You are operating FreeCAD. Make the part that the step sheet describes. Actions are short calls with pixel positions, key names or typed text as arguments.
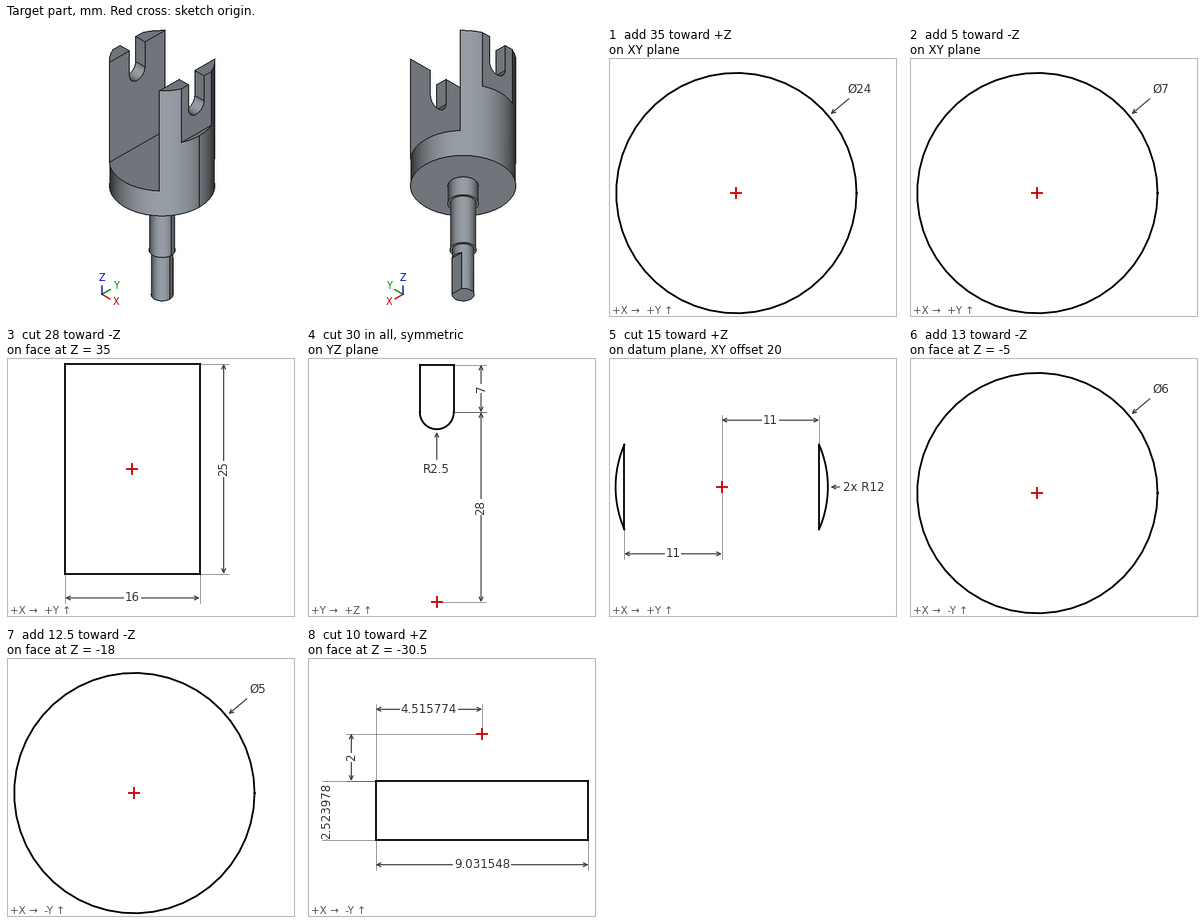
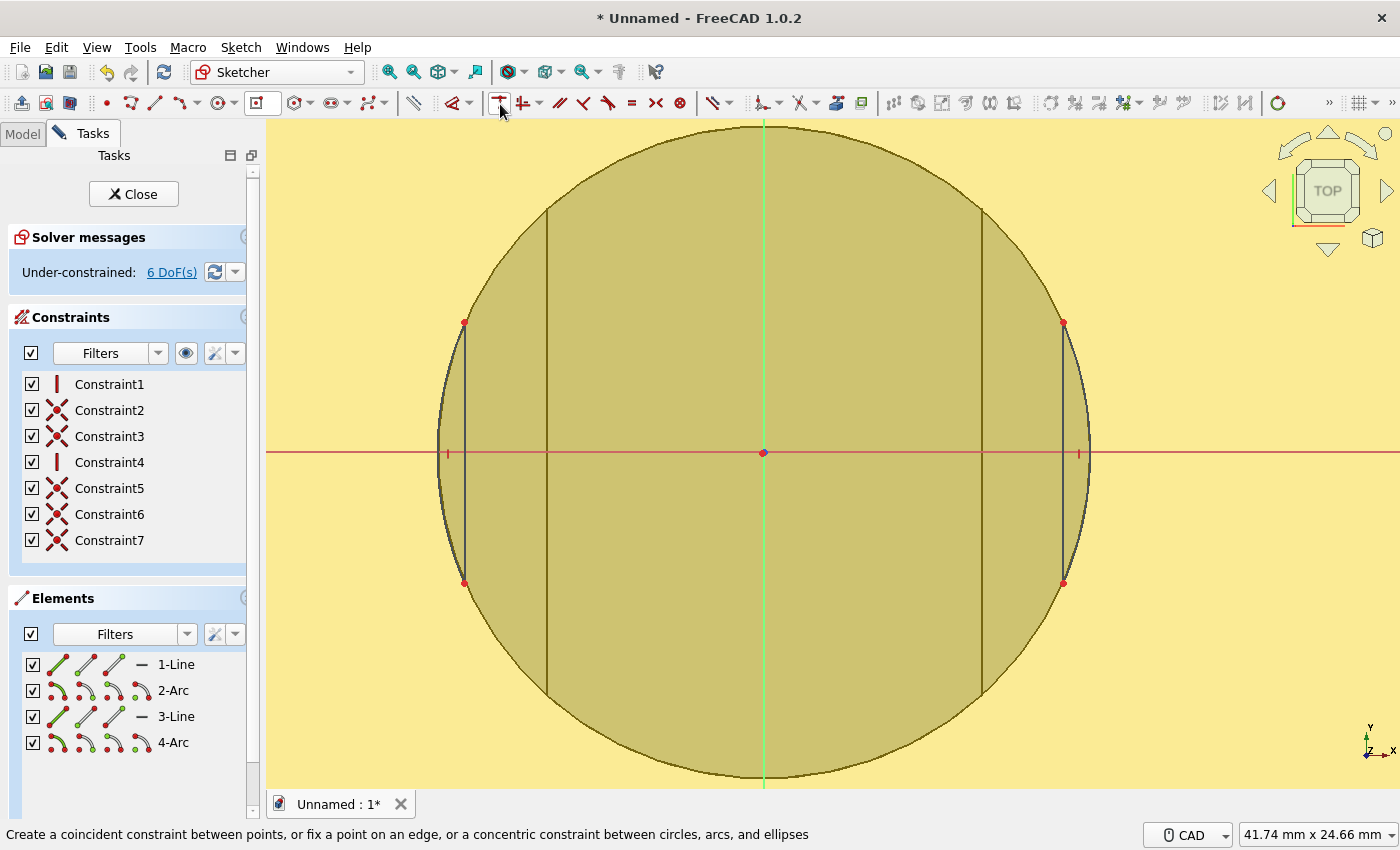
drag(752, 442, 774, 463)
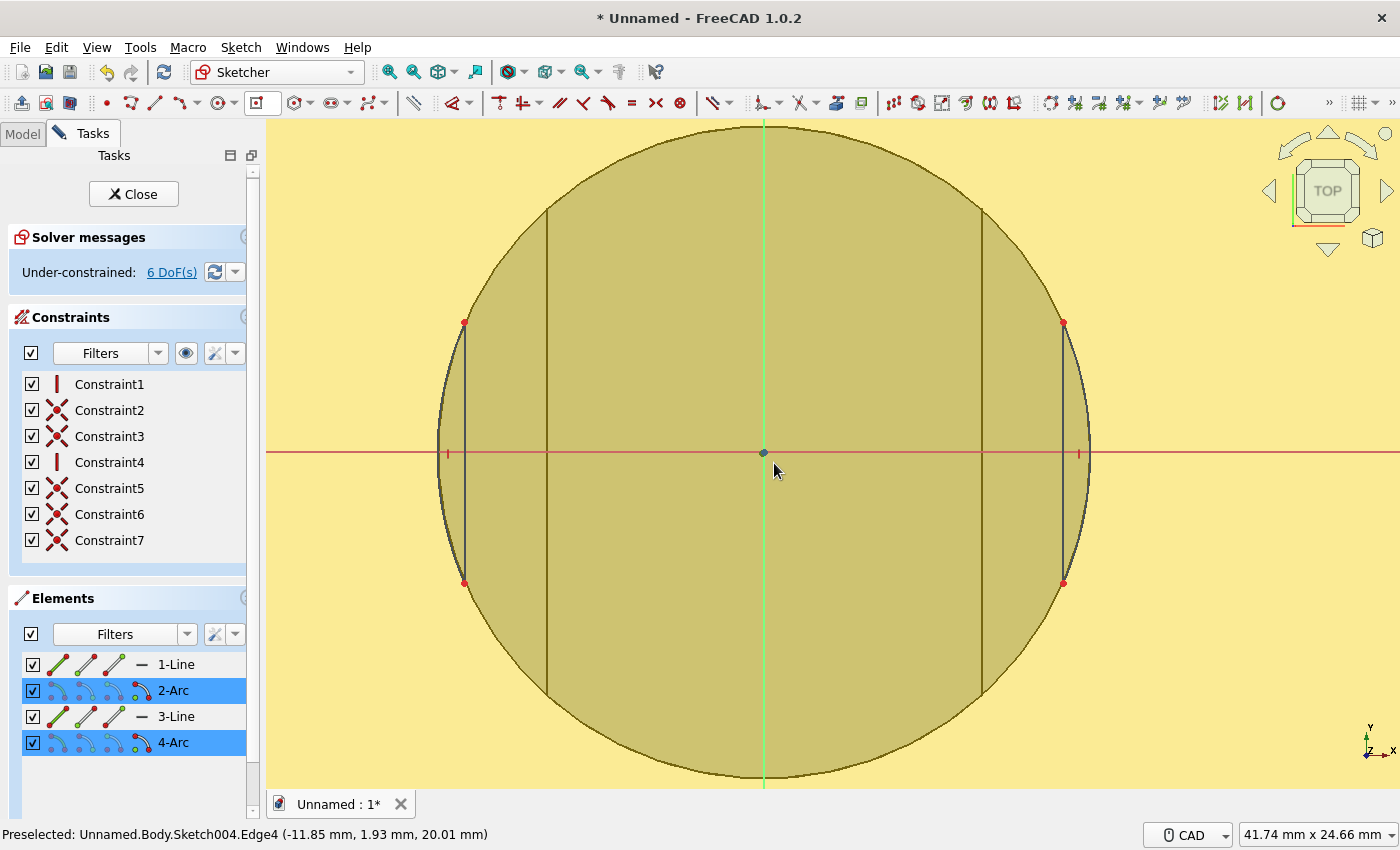
click(500, 104)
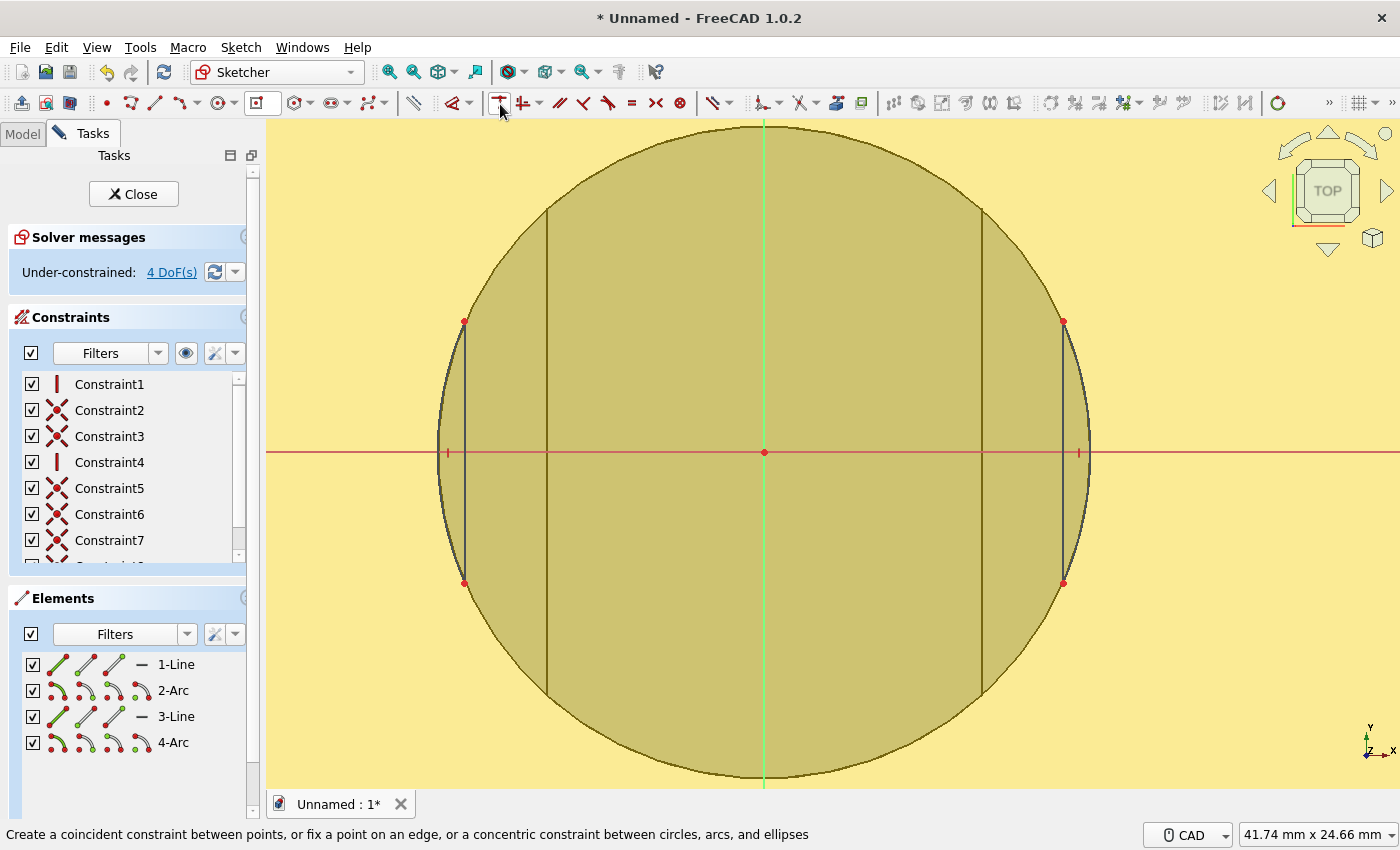
click(1086, 506)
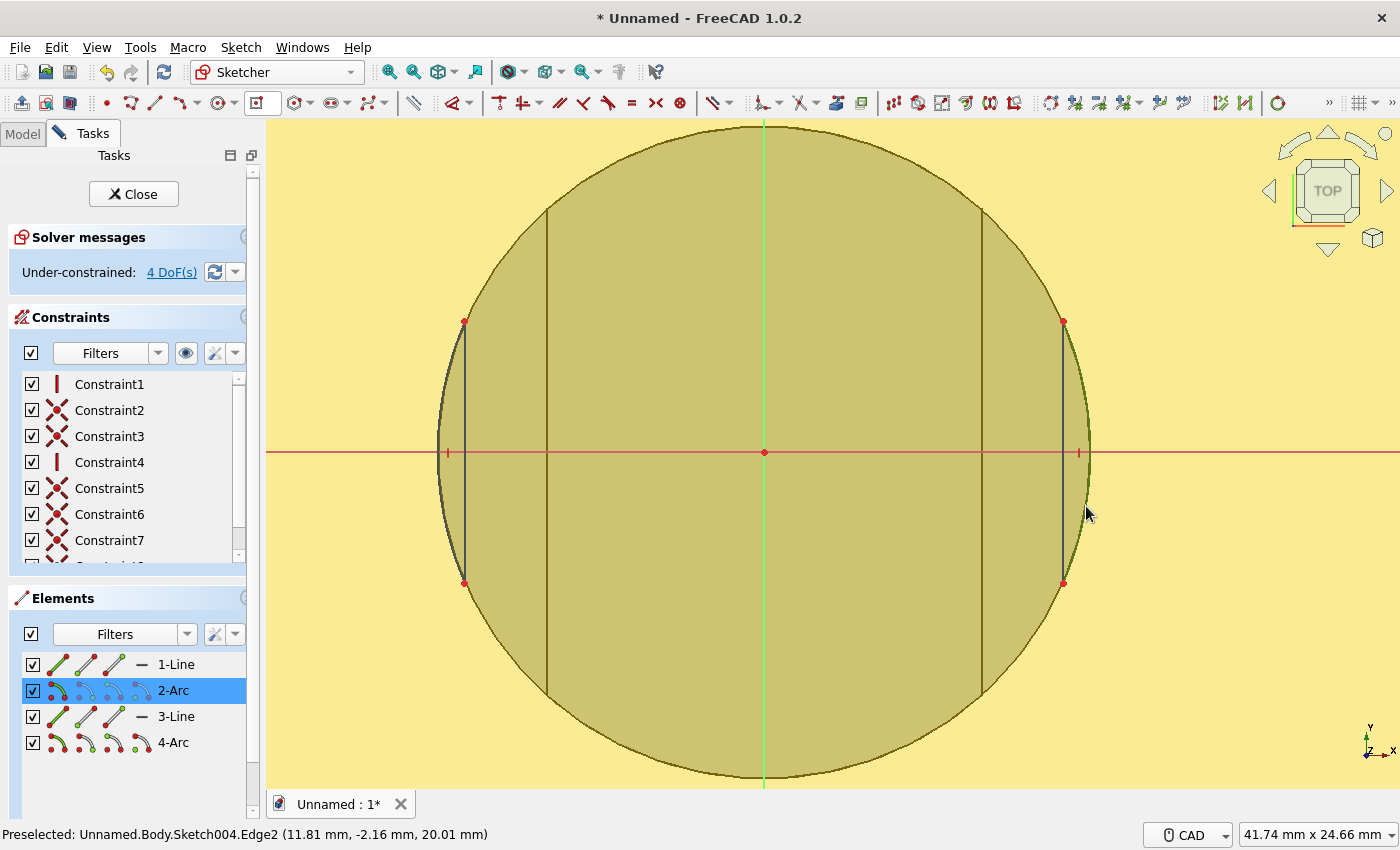
click(442, 399)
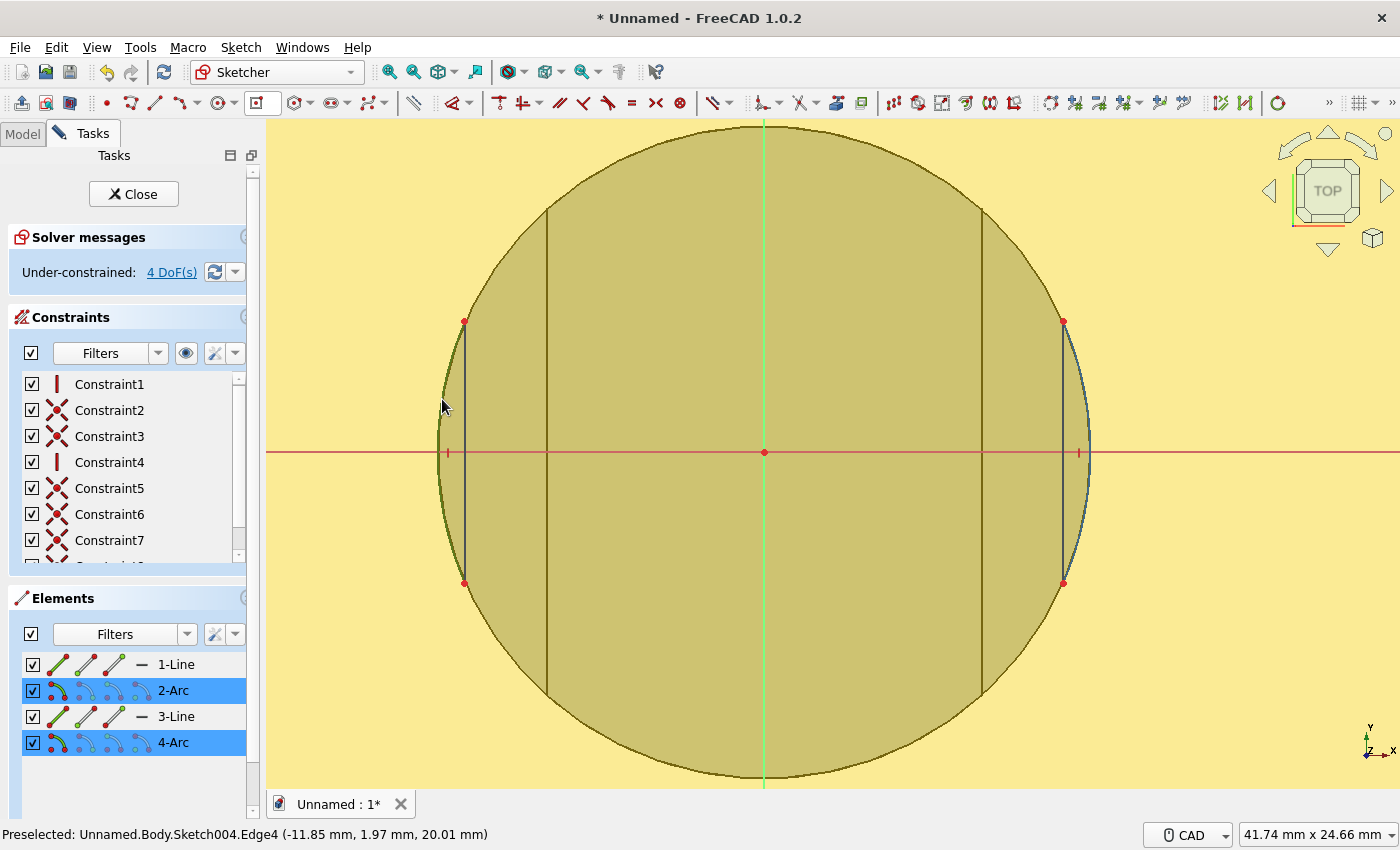
click(632, 104)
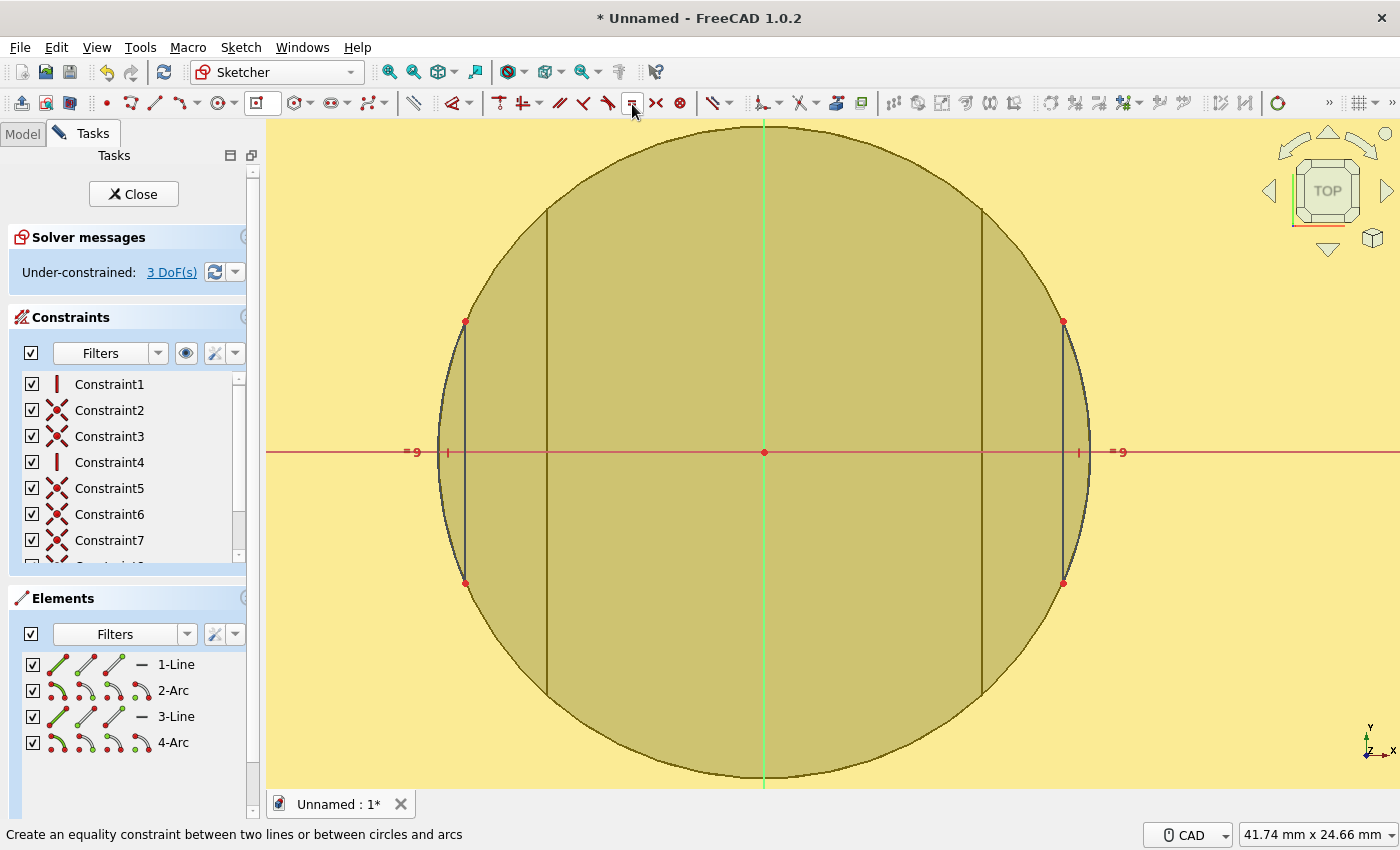
click(452, 104)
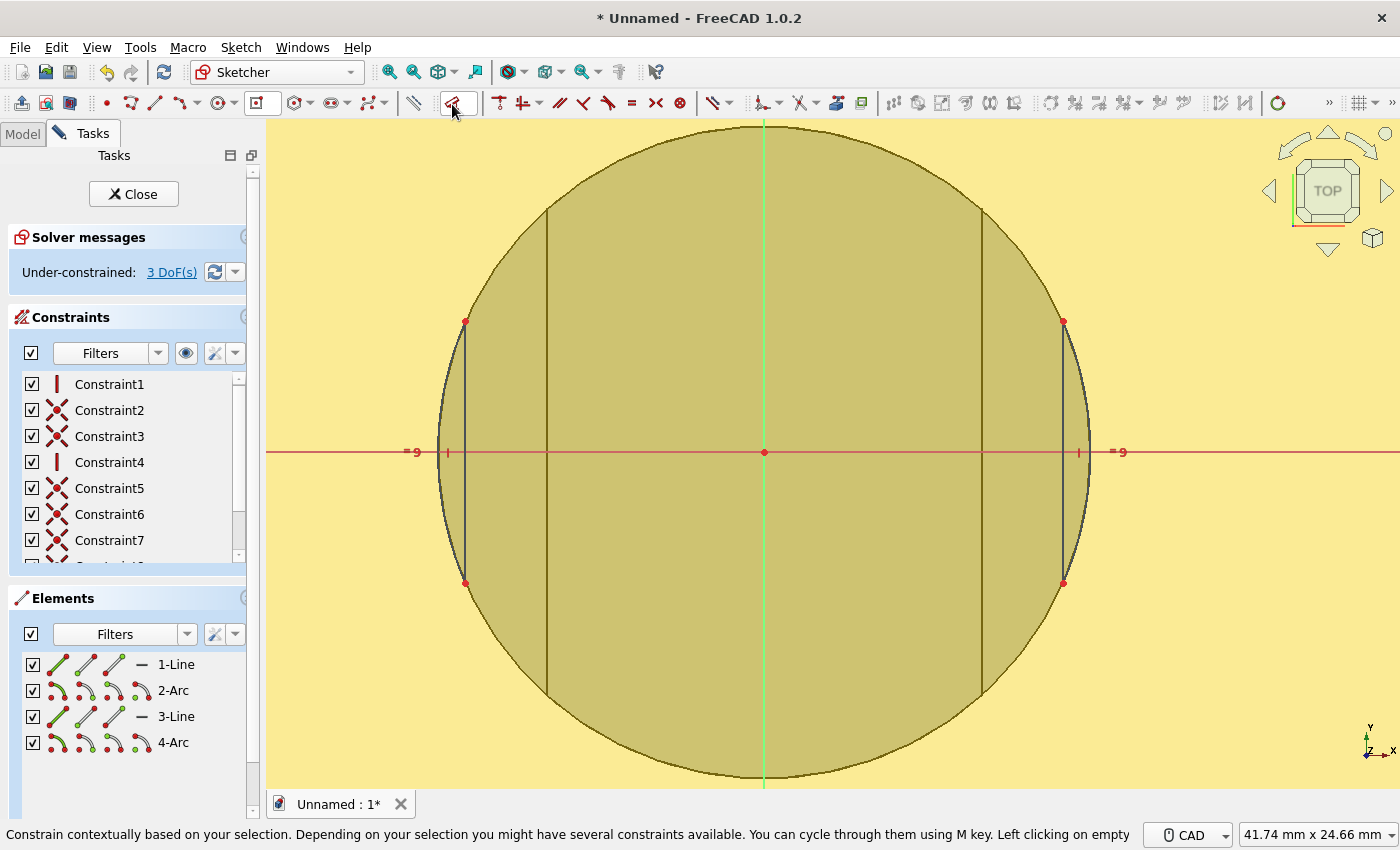
click(1086, 506)
click(1118, 511)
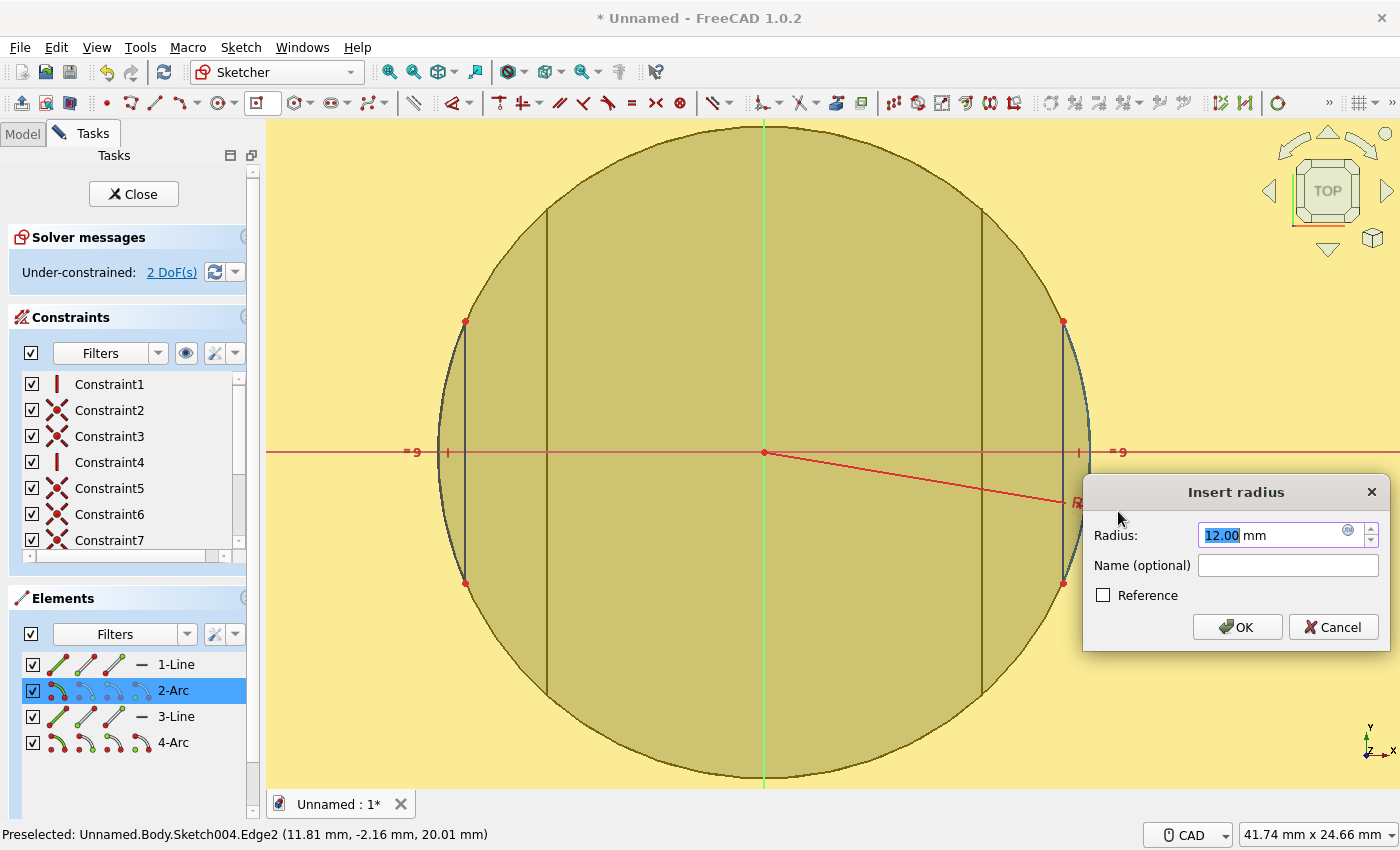
text(12)
key(Return)